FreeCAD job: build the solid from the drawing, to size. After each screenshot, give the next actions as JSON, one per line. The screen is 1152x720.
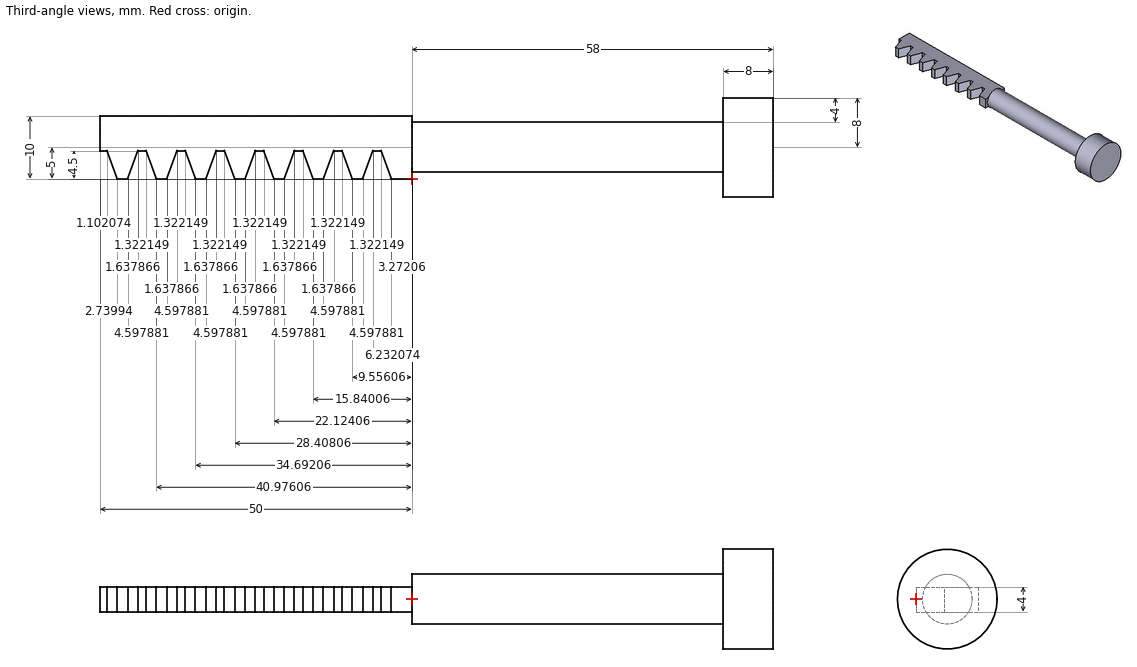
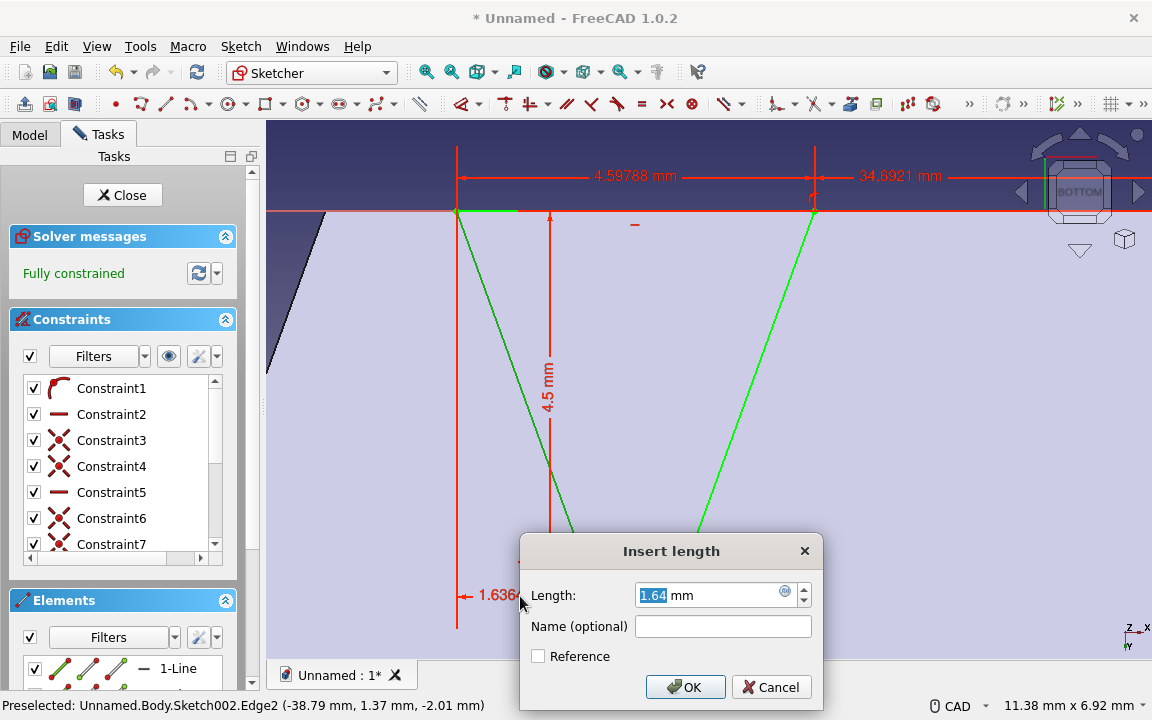
{"action": "type", "text": "1.637866"}
{"action": "key", "text": "Return"}
{"action": "key", "text": "Escape"}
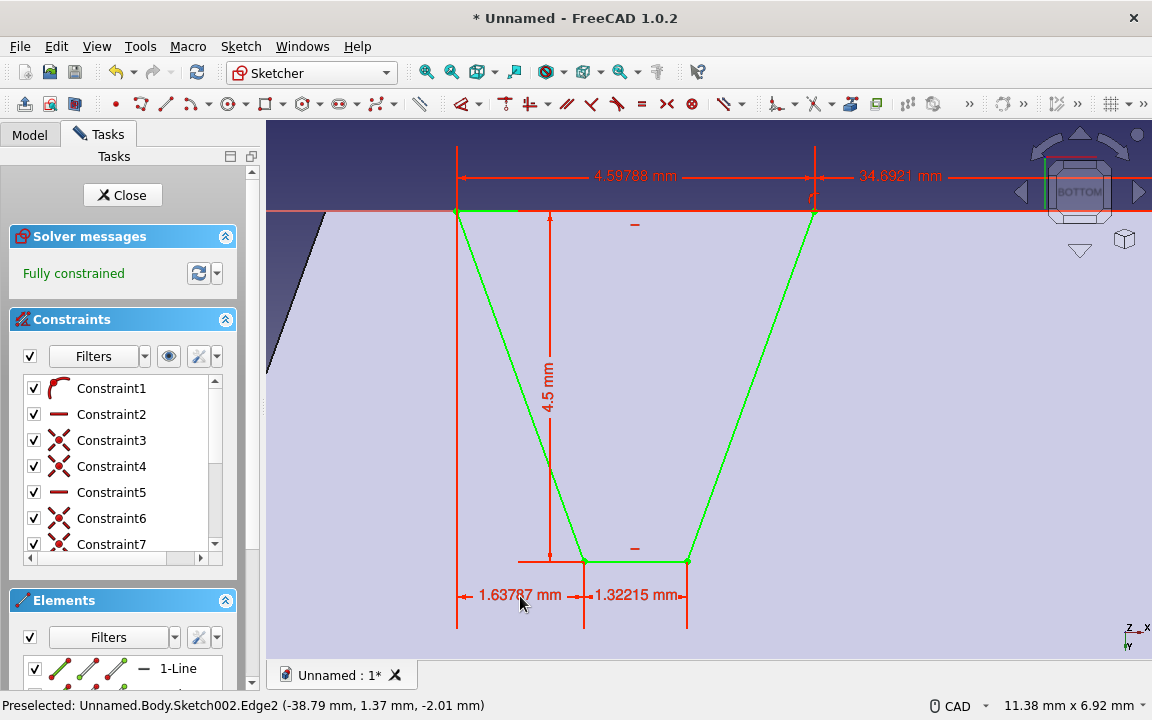
{"action": "left_click", "coordinate": [123, 195]}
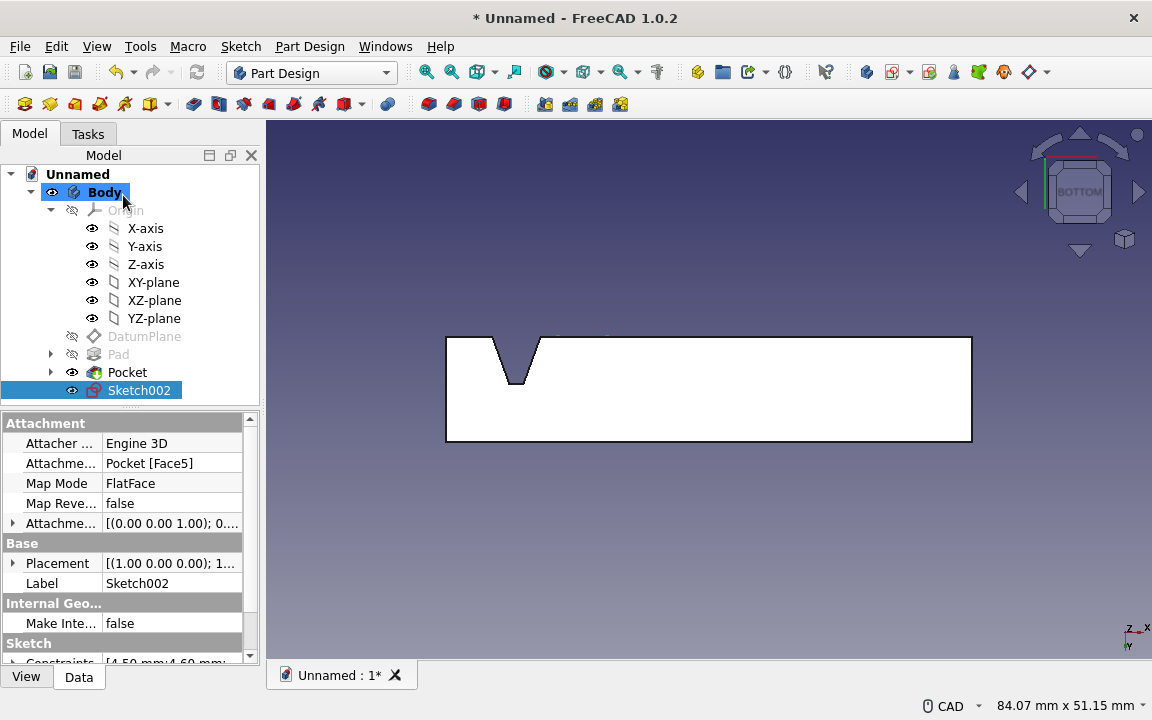
{"action": "left_click", "coordinate": [194, 104]}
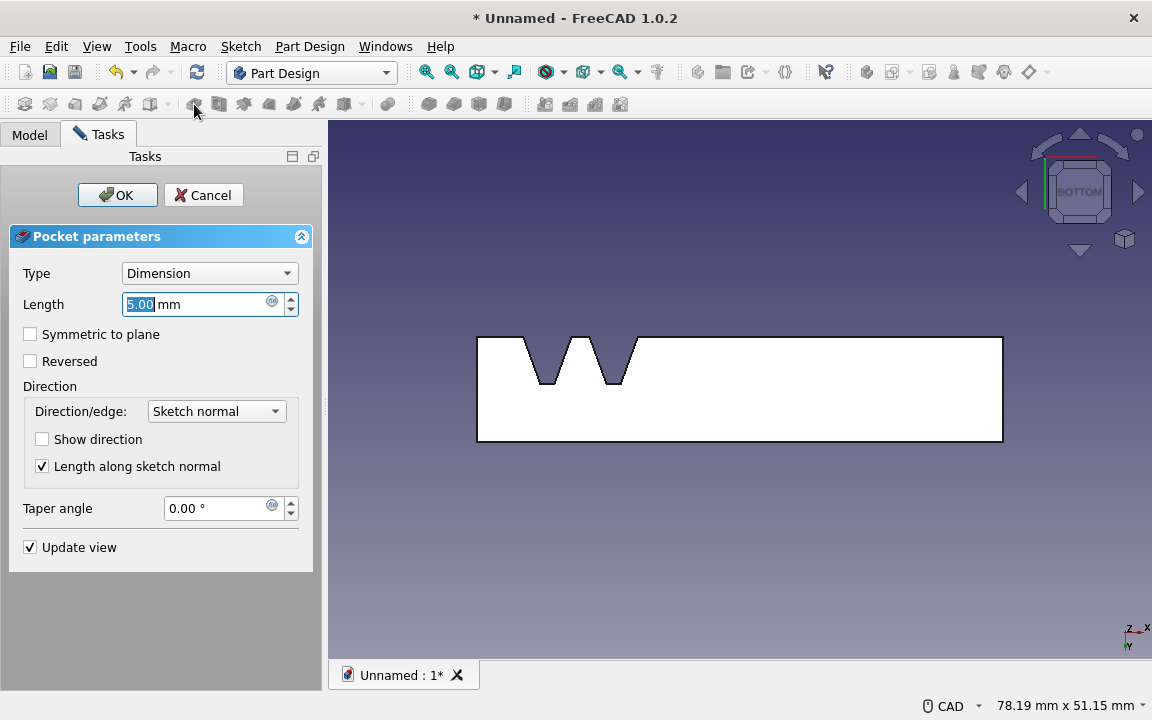
{"action": "left_click", "coordinate": [210, 274]}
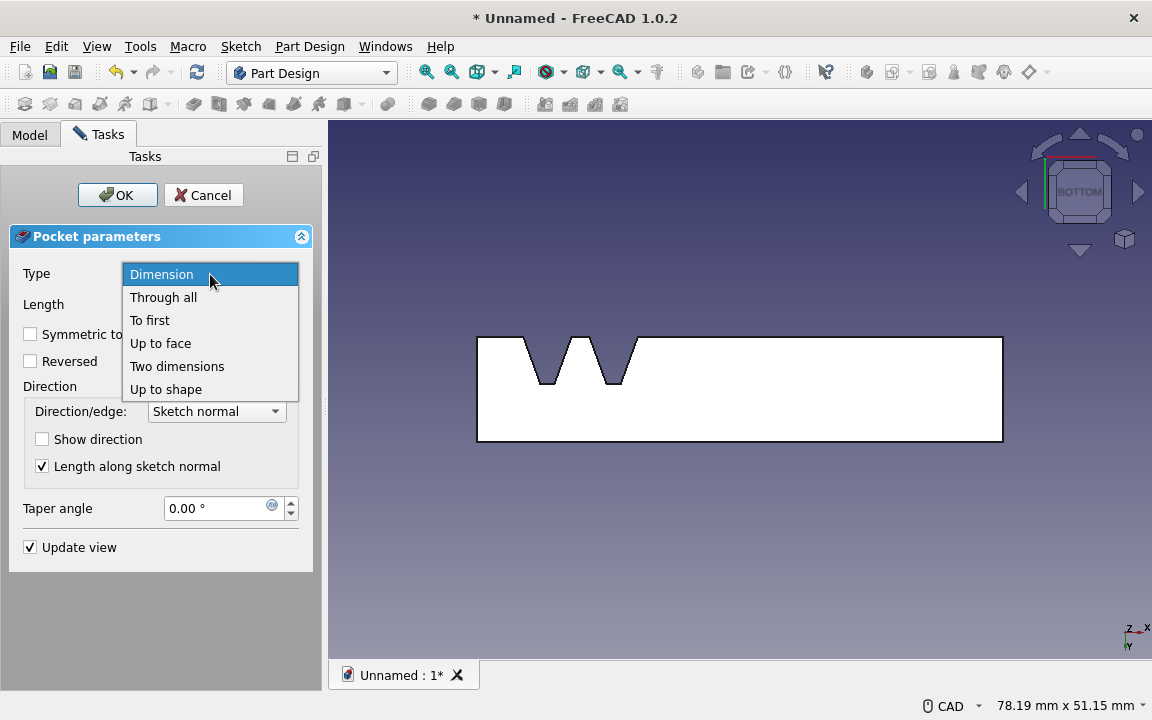
{"action": "left_click", "coordinate": [208, 298]}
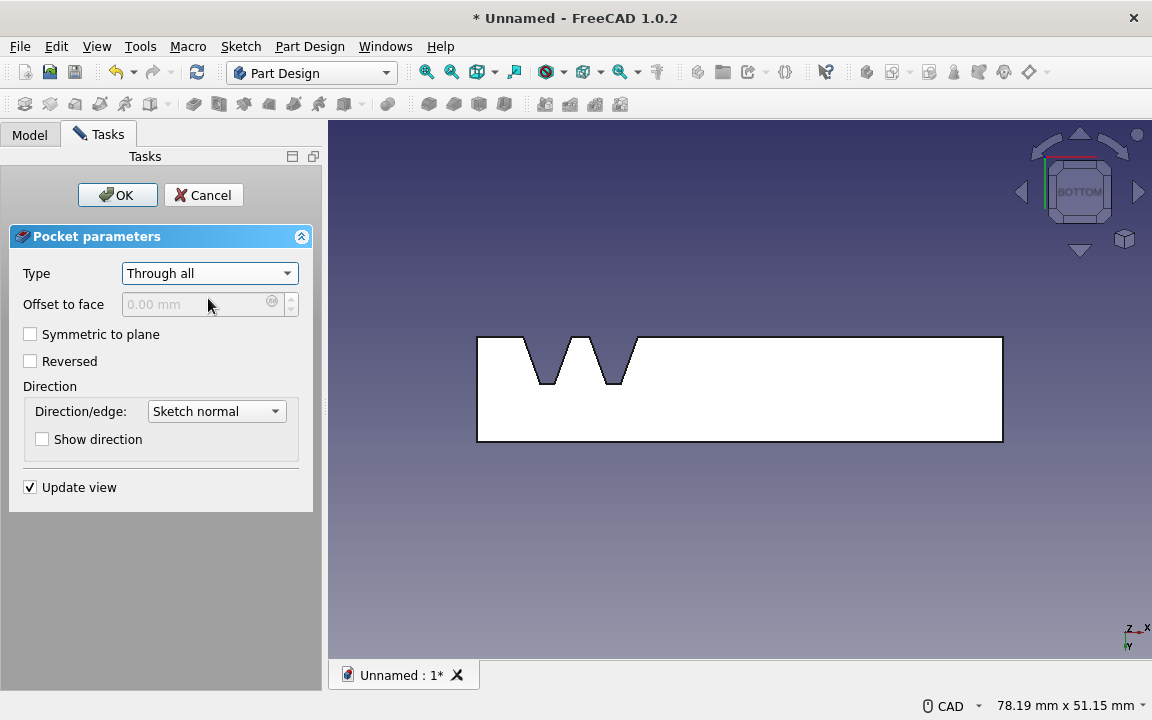
{"action": "left_click", "coordinate": [118, 195]}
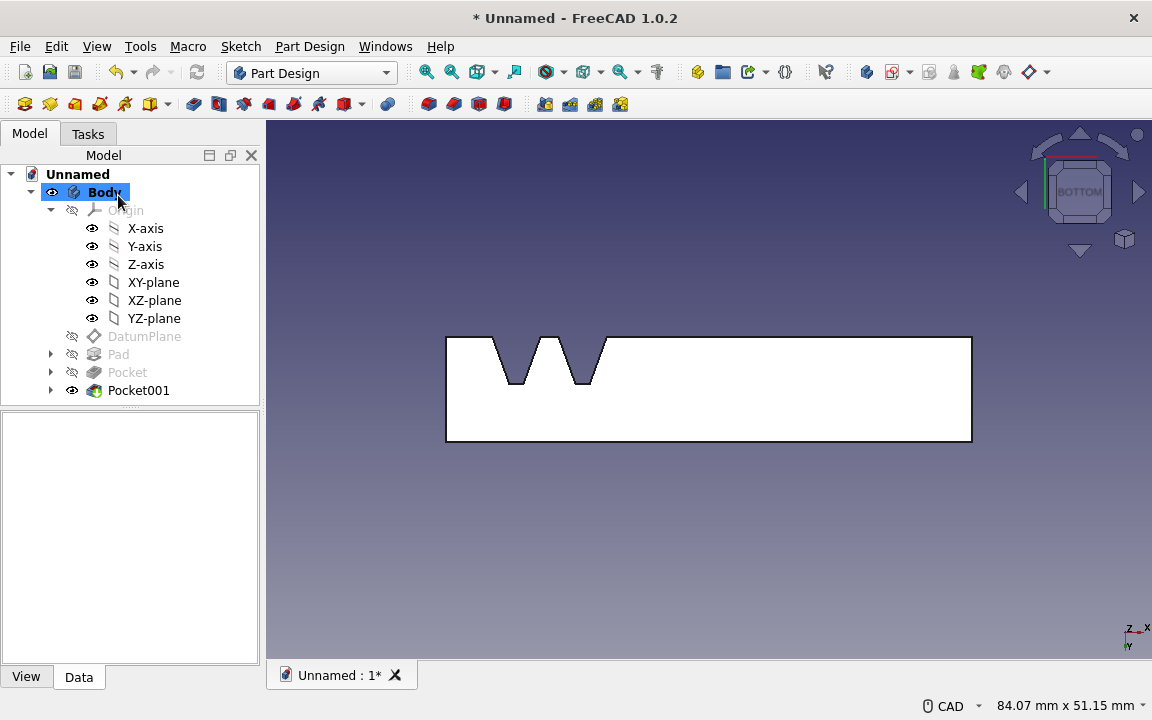
{"action": "left_click", "coordinate": [860, 389]}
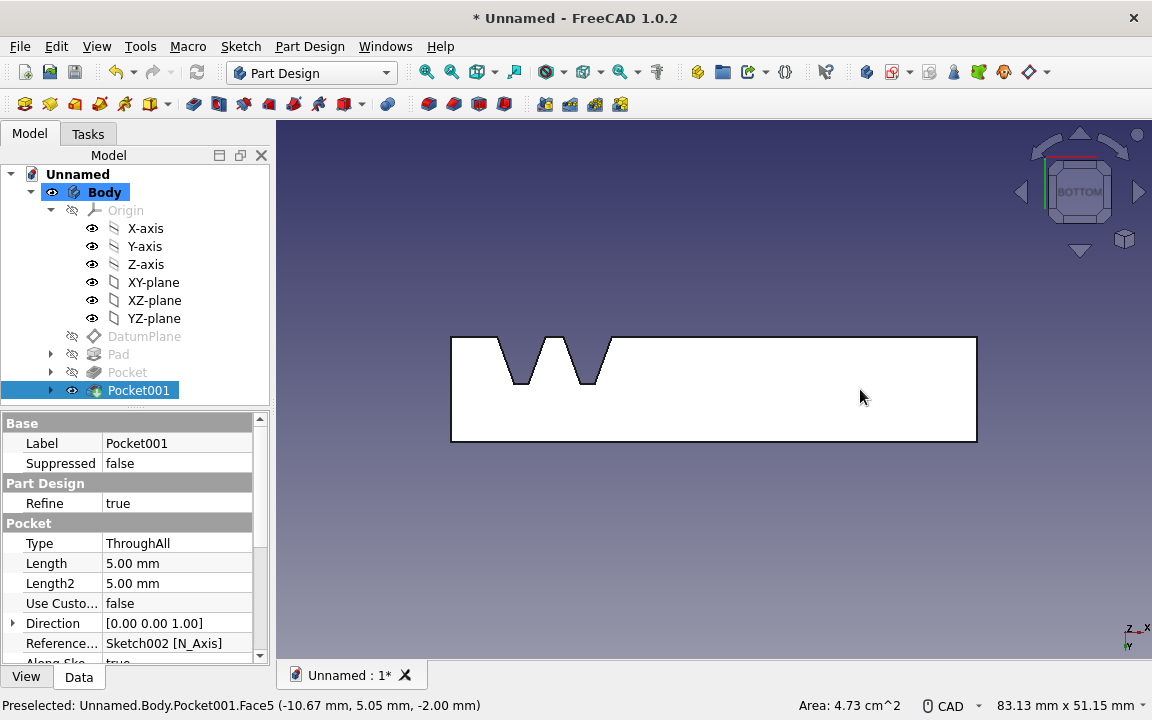
{"action": "left_click", "coordinate": [892, 72]}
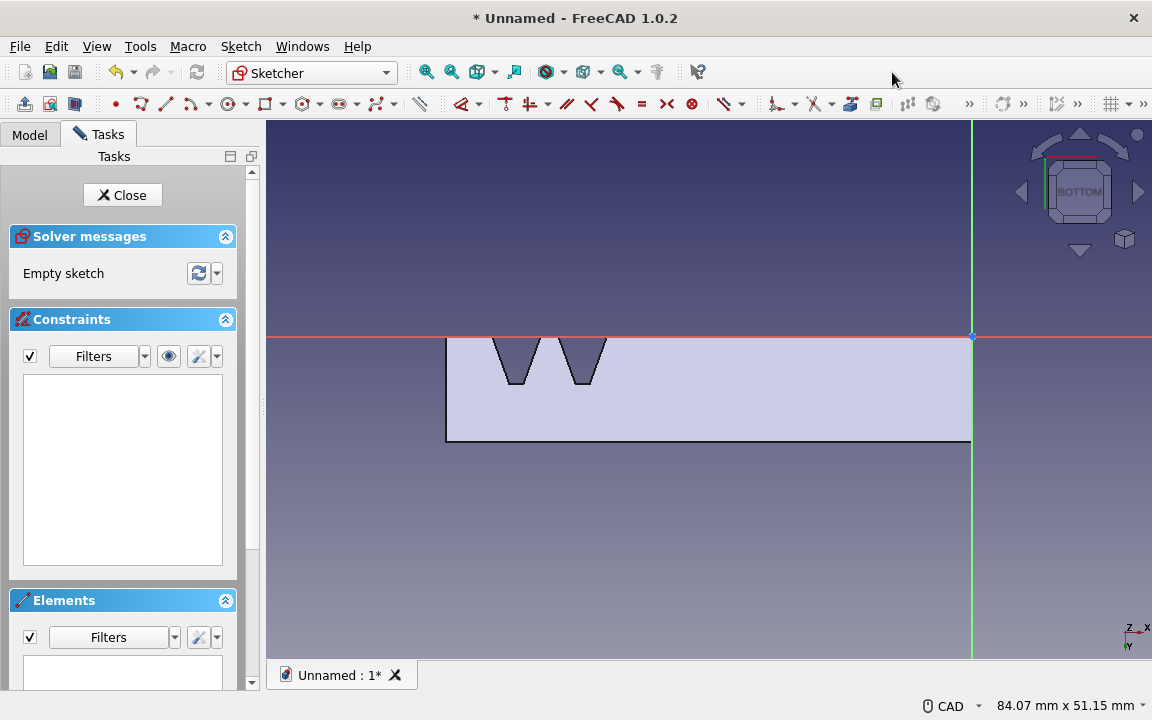
{"action": "scroll", "coordinate": [650, 356], "scroll_direction": "up", "scroll_amount": 10}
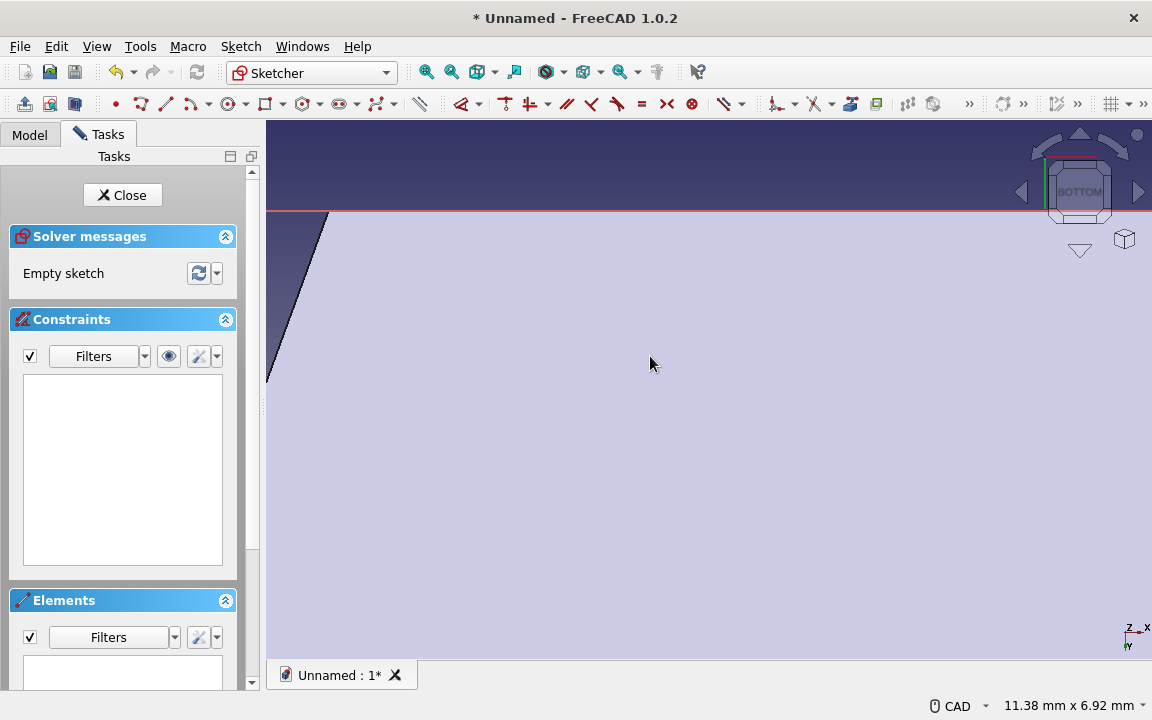
{"action": "left_click", "coordinate": [141, 104]}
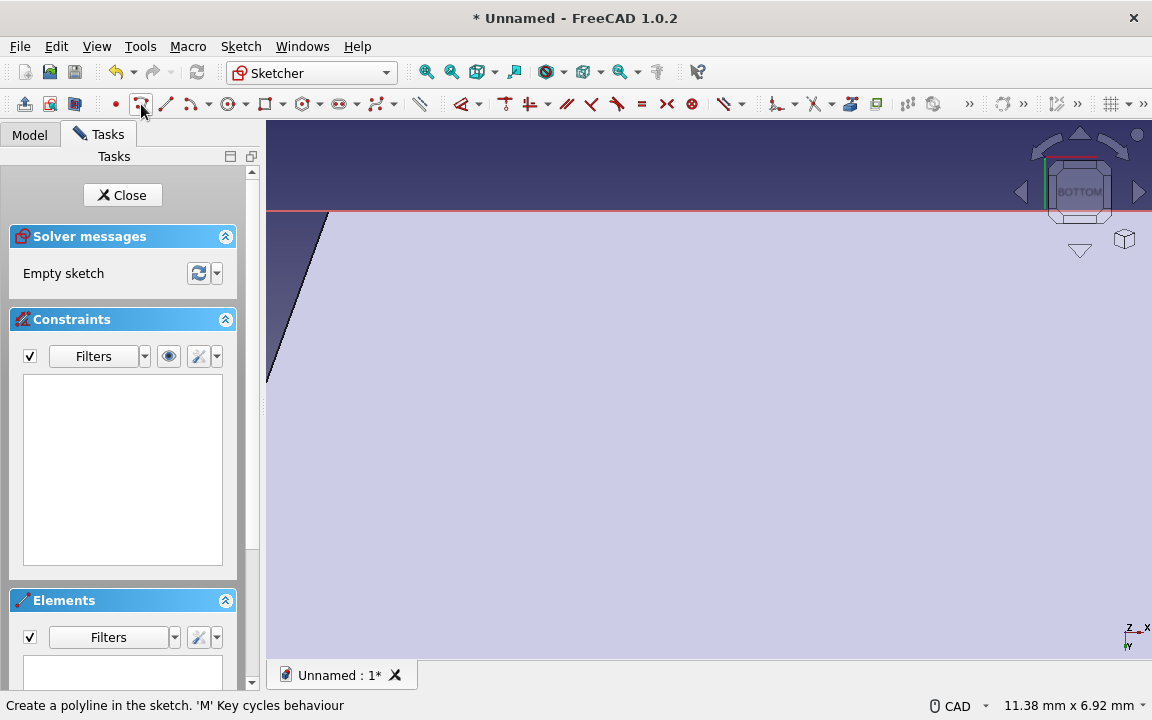
{"action": "left_click", "coordinate": [818, 211]}
{"action": "left_click", "coordinate": [460, 220]}
{"action": "left_click", "coordinate": [587, 562]}
{"action": "left_click", "coordinate": [690, 562]}
{"action": "left_click", "coordinate": [818, 211]}
{"action": "key", "text": "Escape"}
{"action": "key", "text": "Escape"}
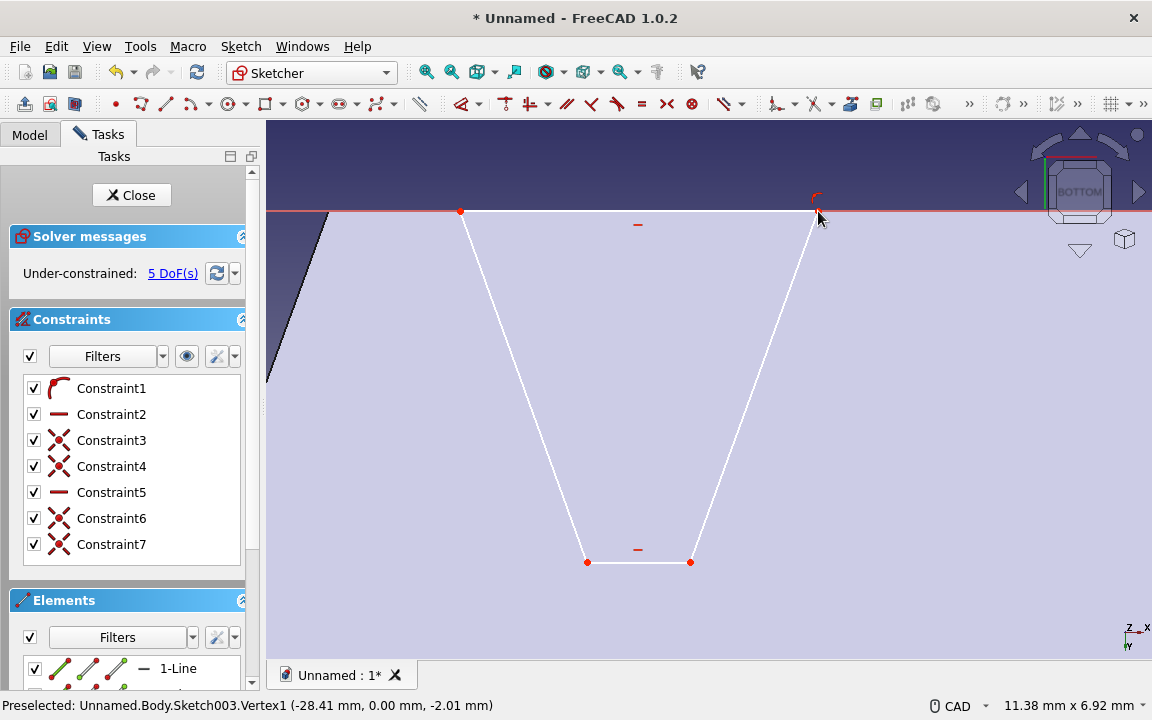
{"action": "left_click", "coordinate": [460, 104]}